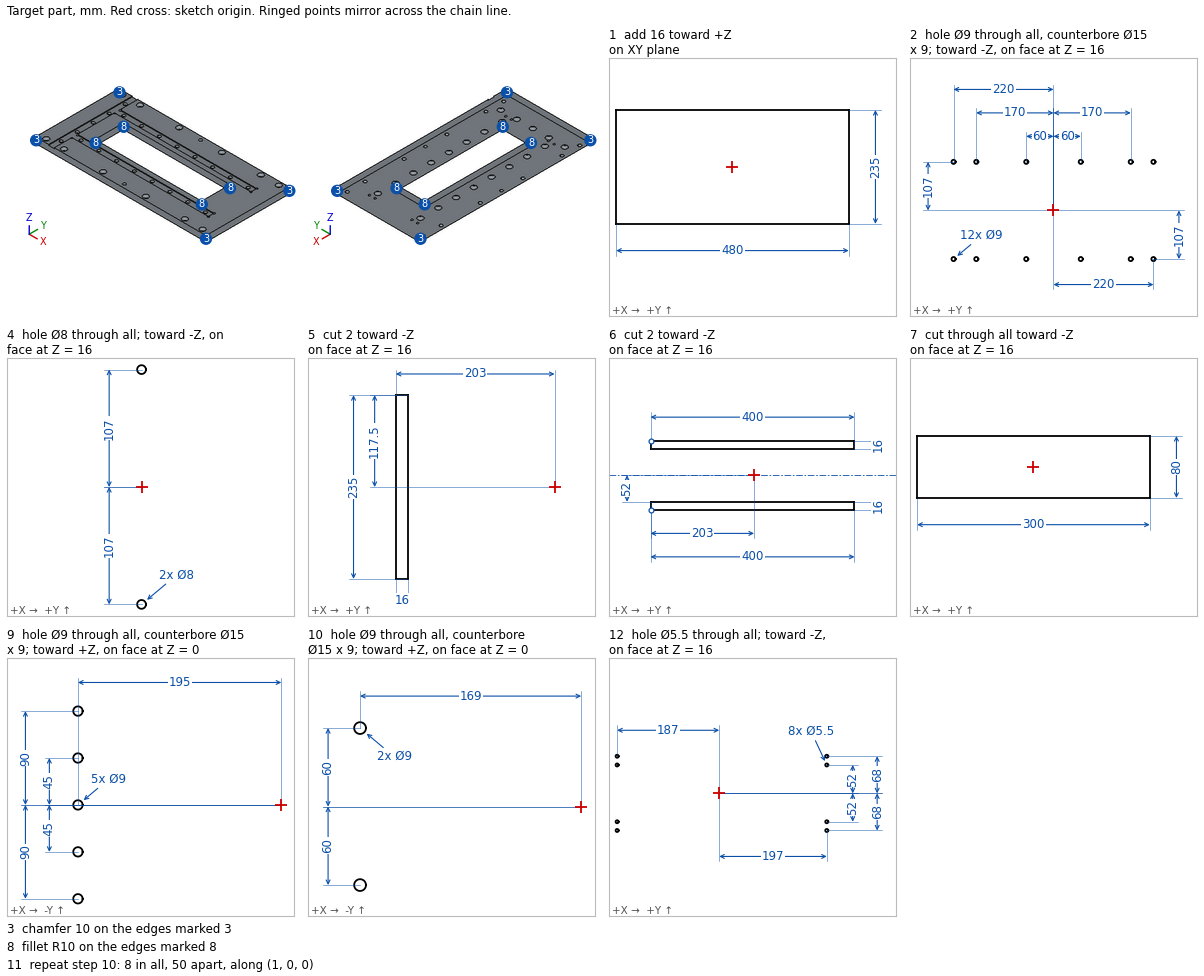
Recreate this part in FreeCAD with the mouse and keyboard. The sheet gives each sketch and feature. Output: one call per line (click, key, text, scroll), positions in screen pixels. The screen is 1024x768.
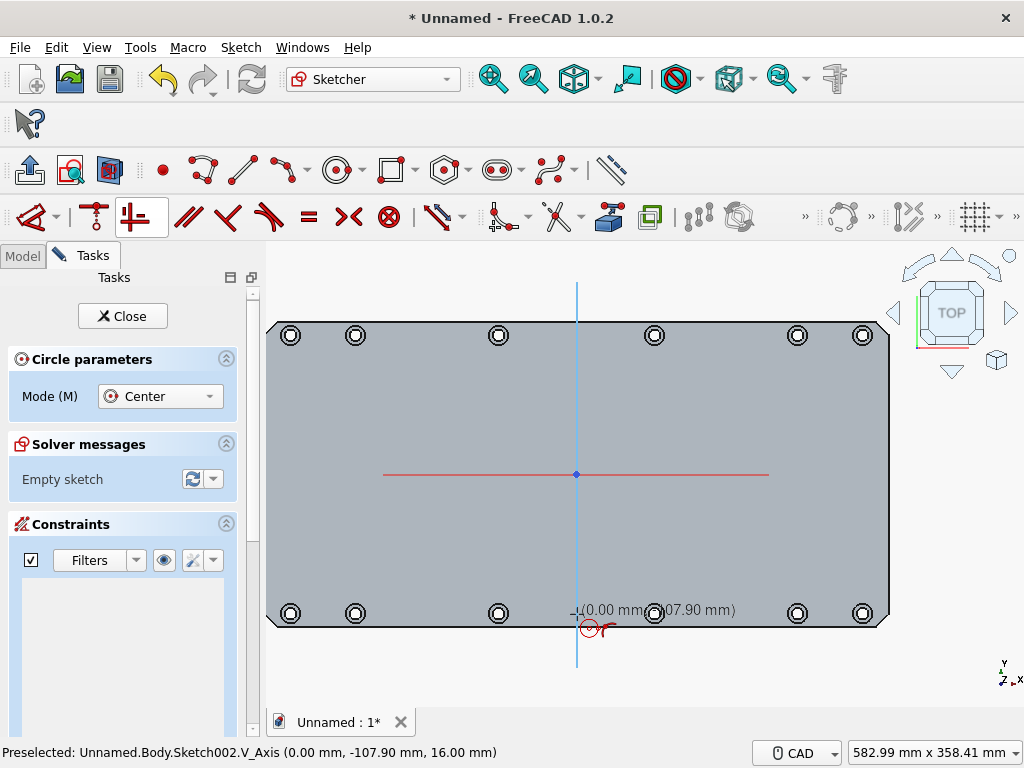
click(577, 614)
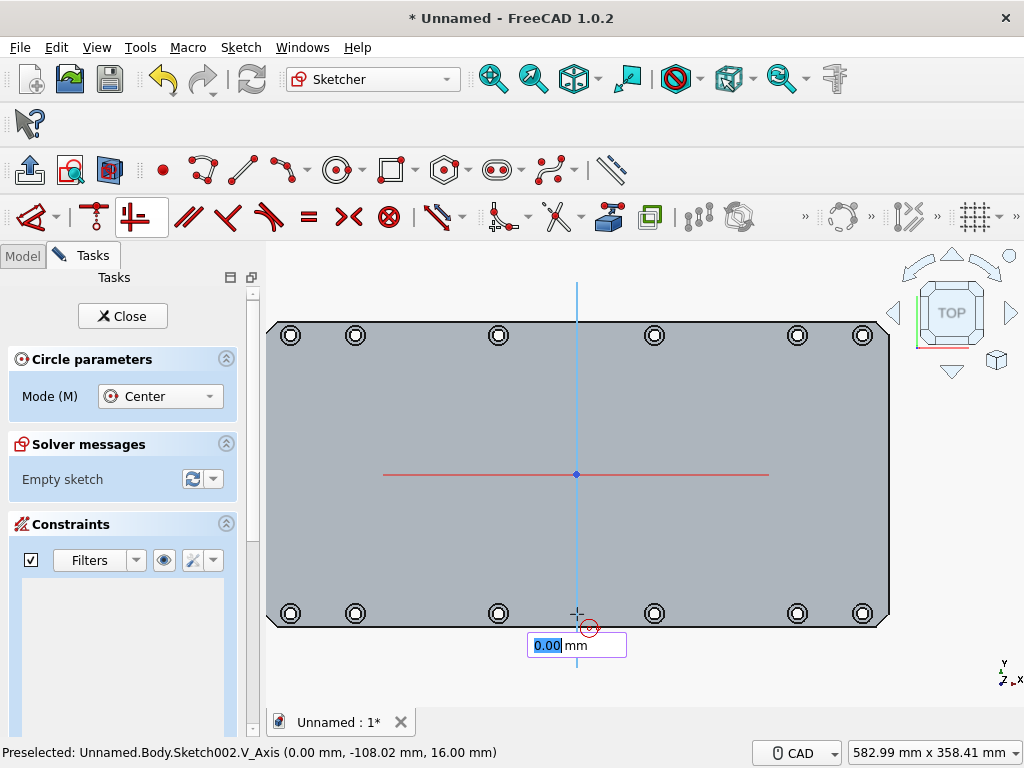
scroll(581, 612, up, 6)
move(582, 610)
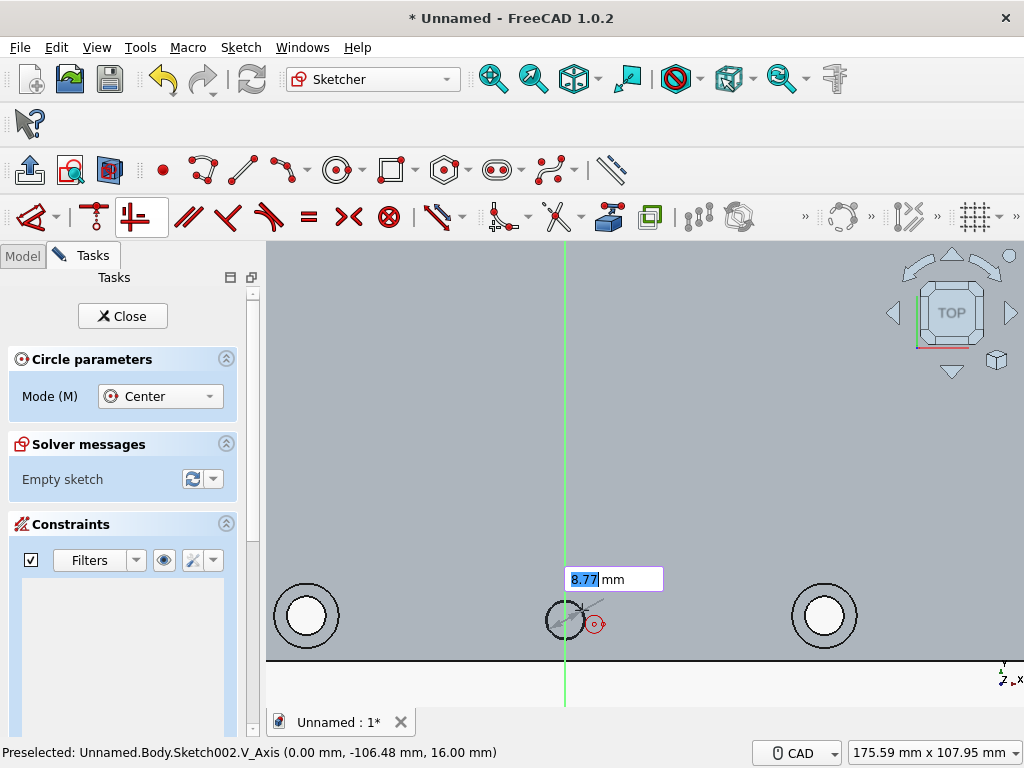
text(8)
key(Return)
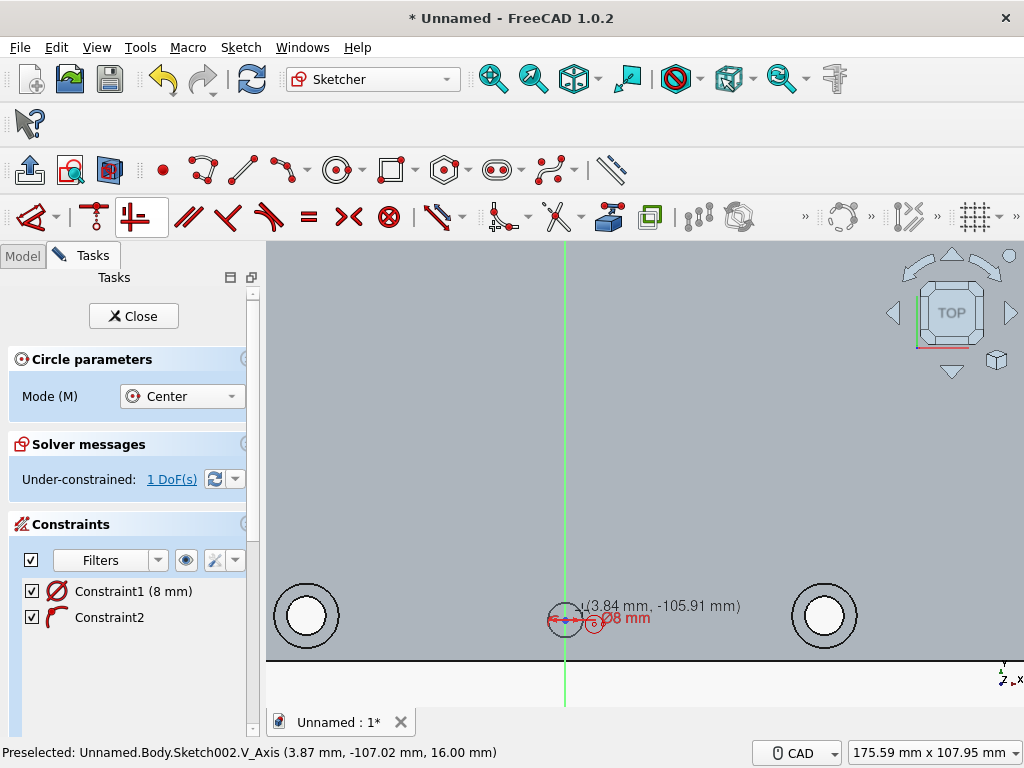
scroll(581, 612, down, 6)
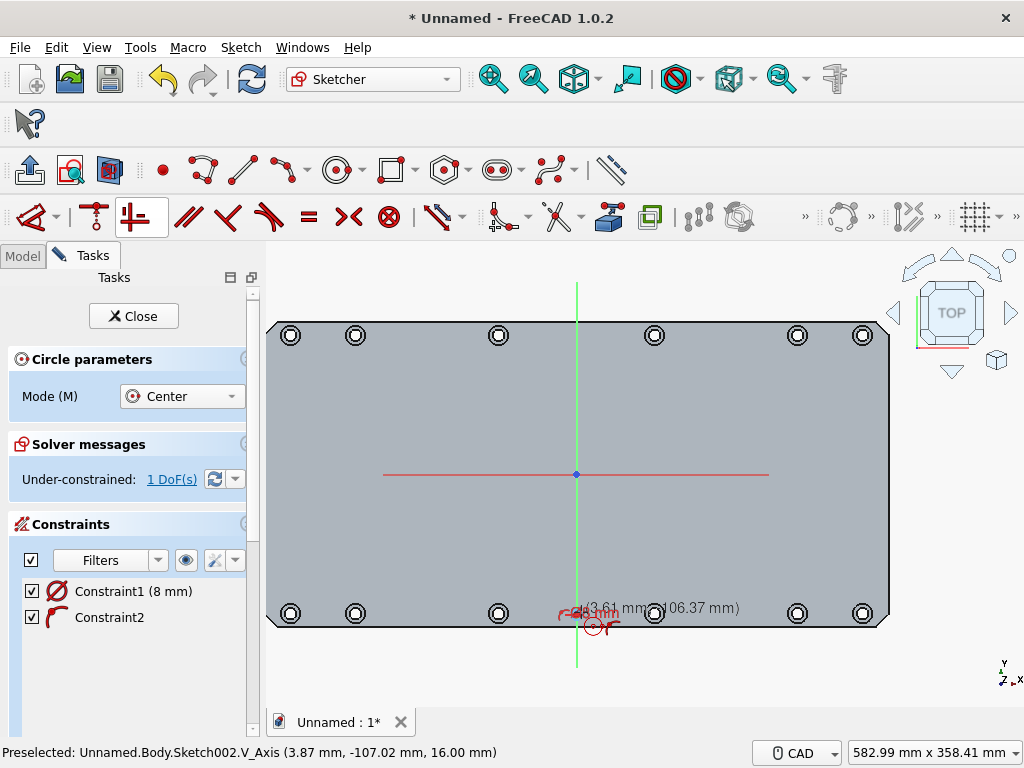
scroll(577, 335, up, 8)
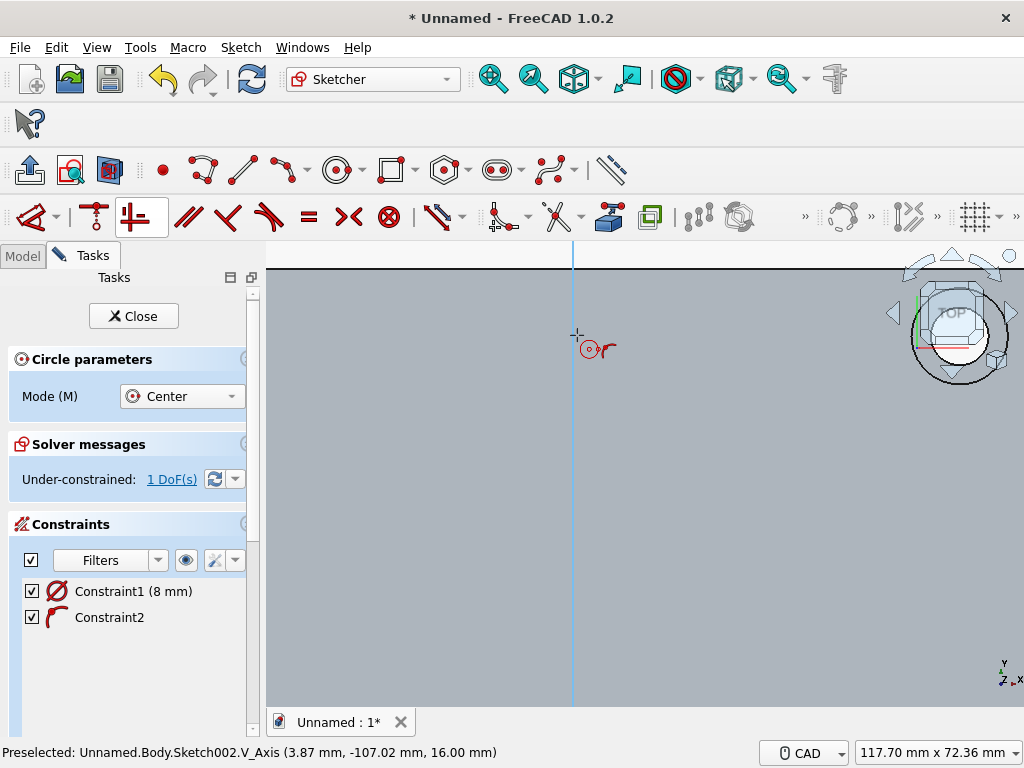
scroll(577, 335, down, 8)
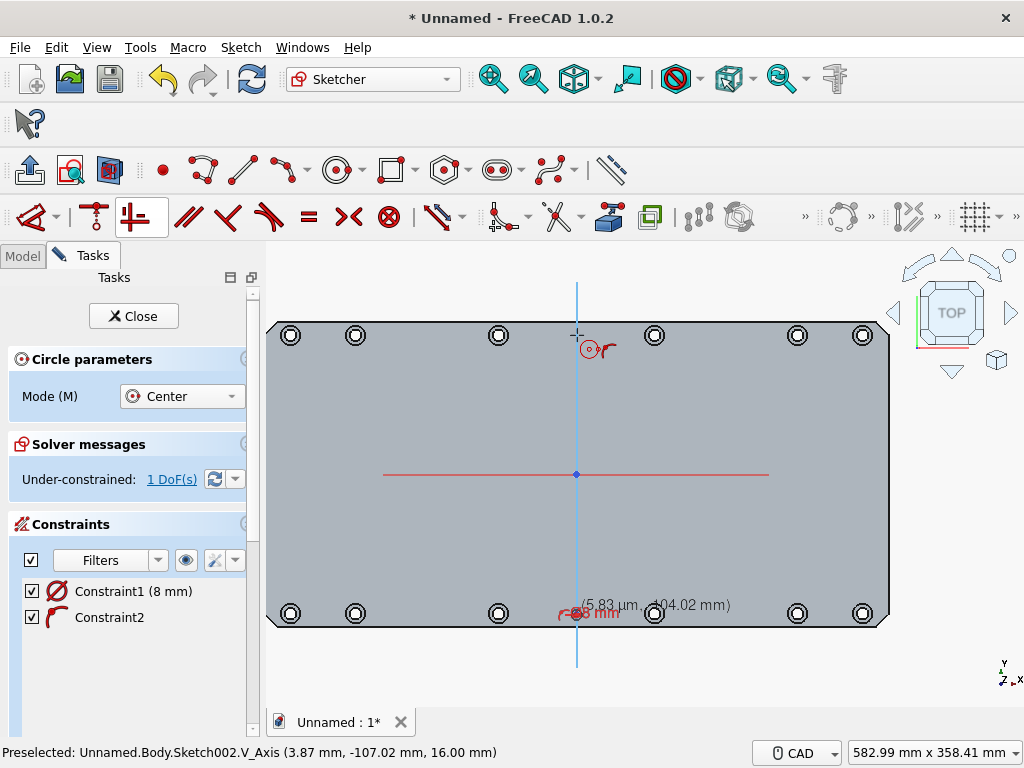
click(577, 335)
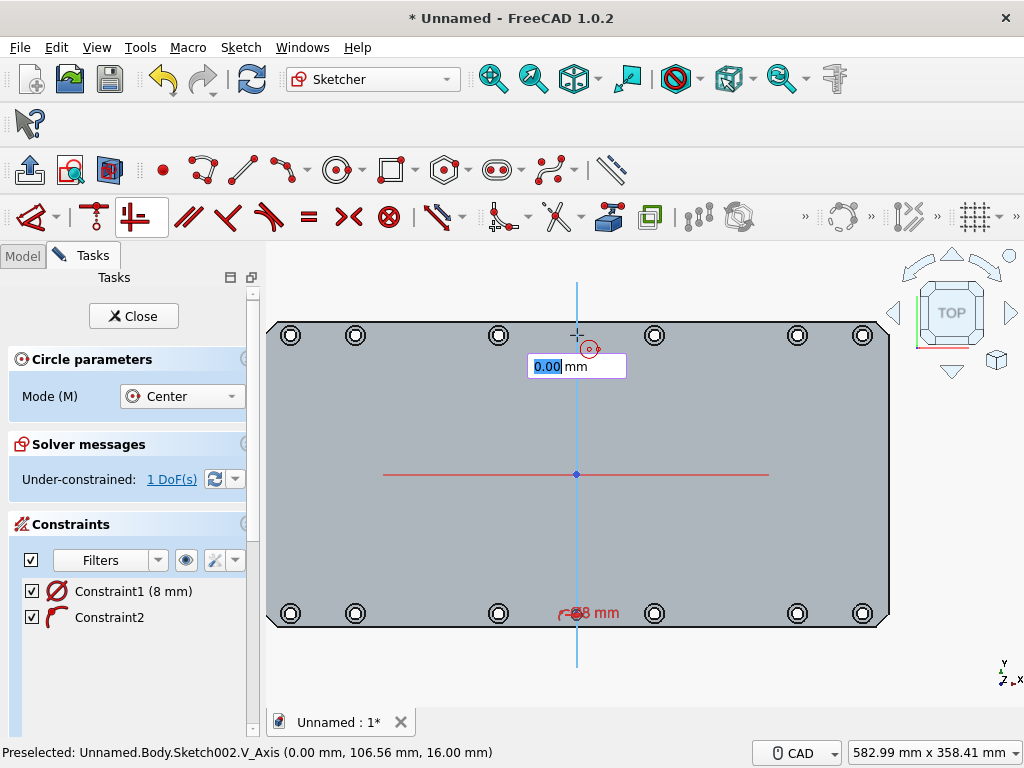
scroll(581, 334, up, 6)
move(582, 332)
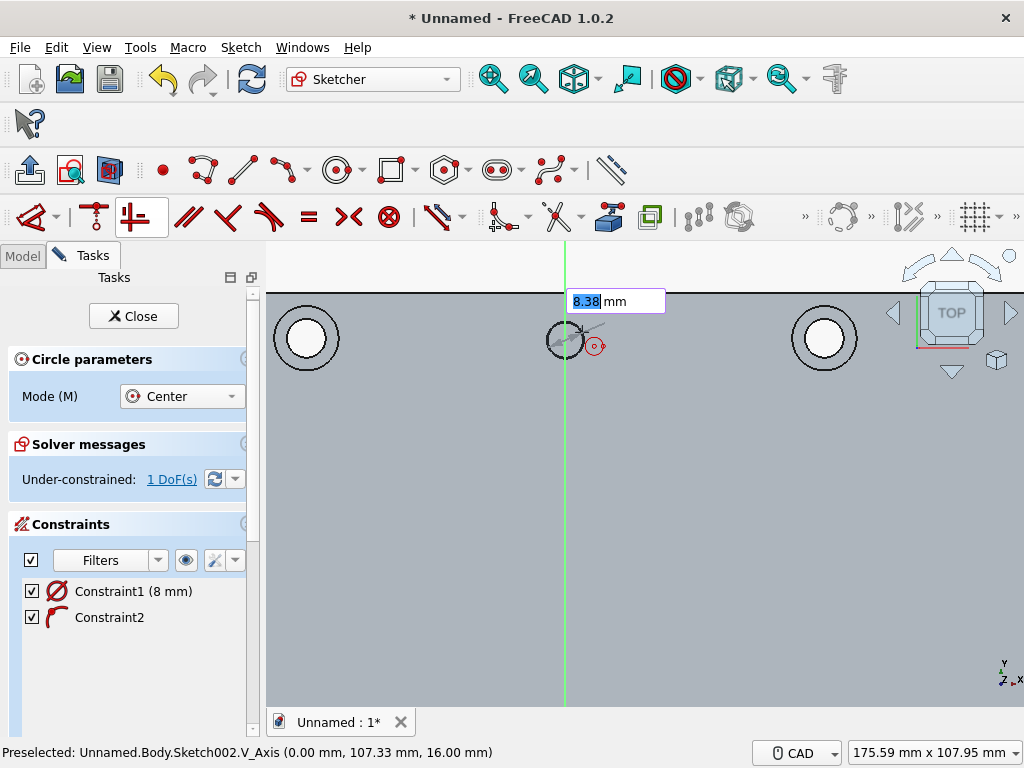
text(8)
key(Return)
key(Escape)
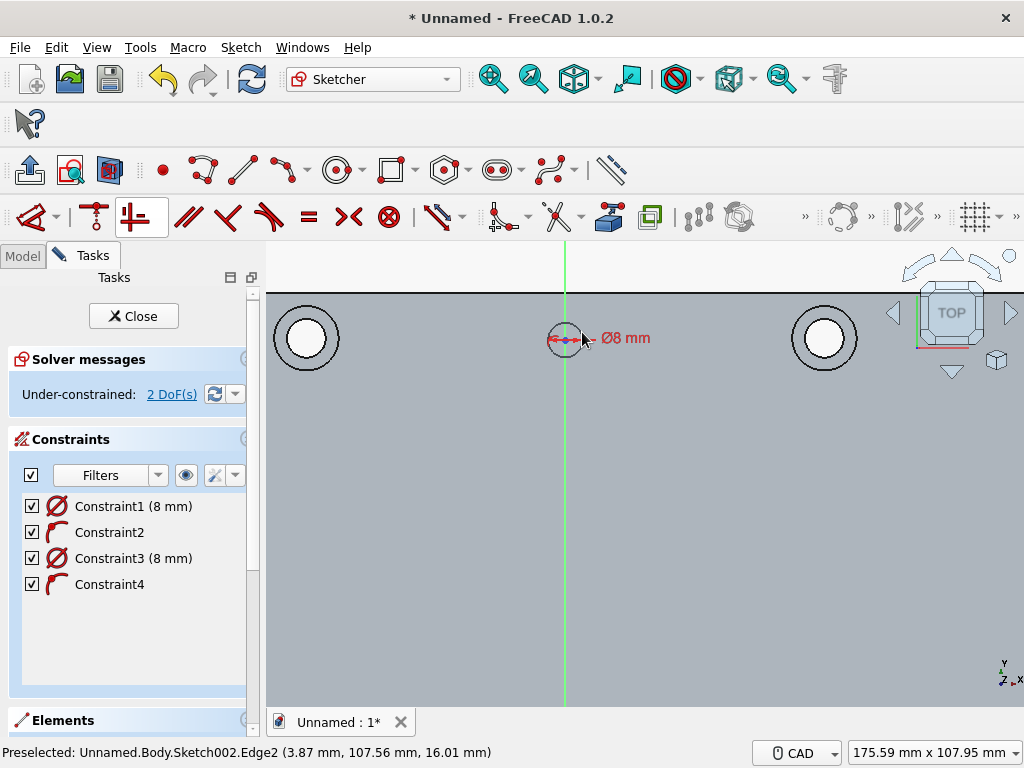
click(32, 218)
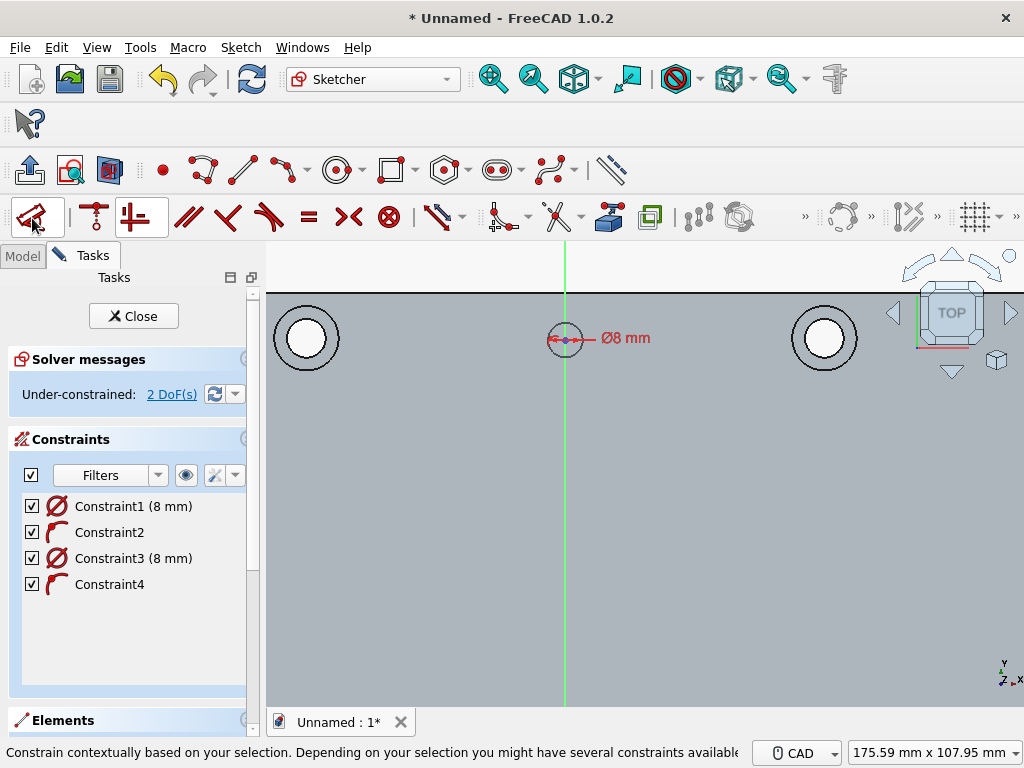
scroll(581, 333, down, 6)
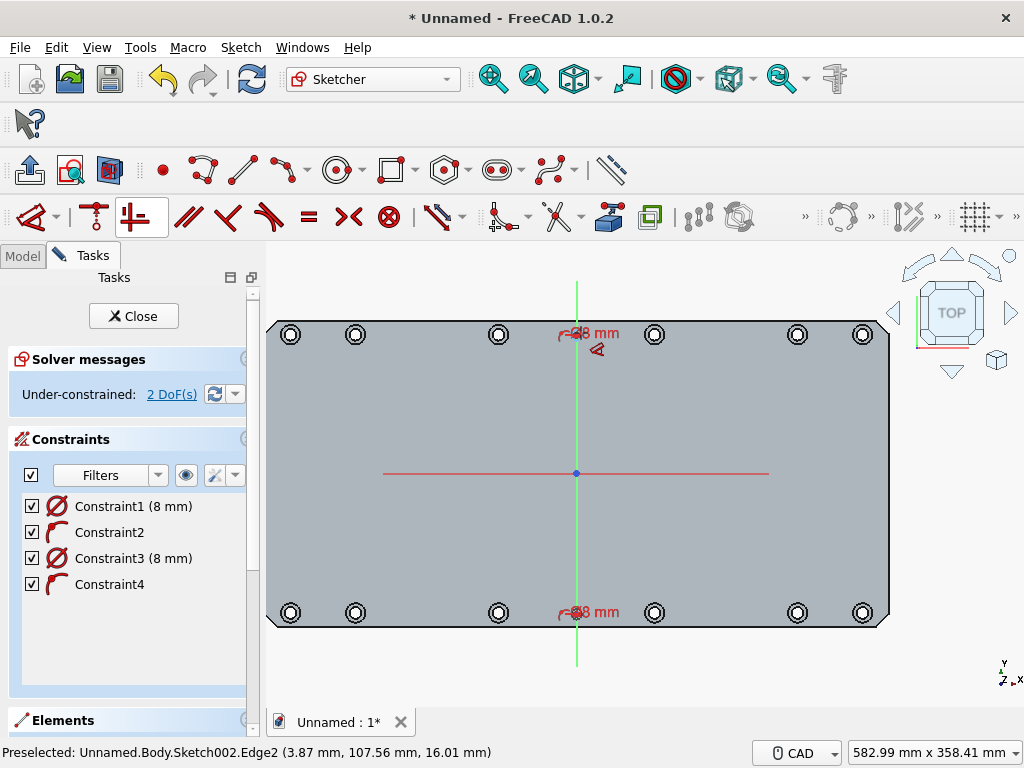
click(577, 614)
click(611, 544)